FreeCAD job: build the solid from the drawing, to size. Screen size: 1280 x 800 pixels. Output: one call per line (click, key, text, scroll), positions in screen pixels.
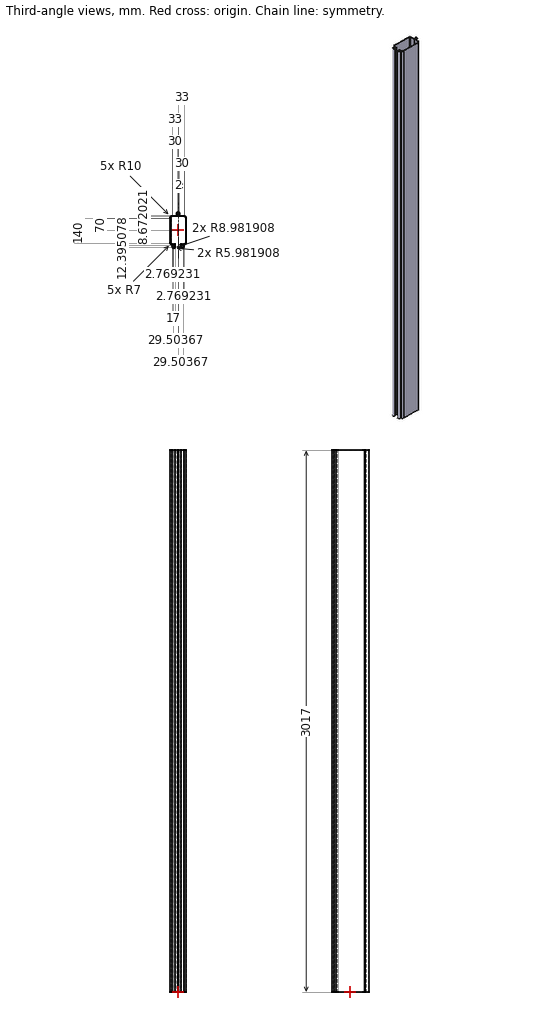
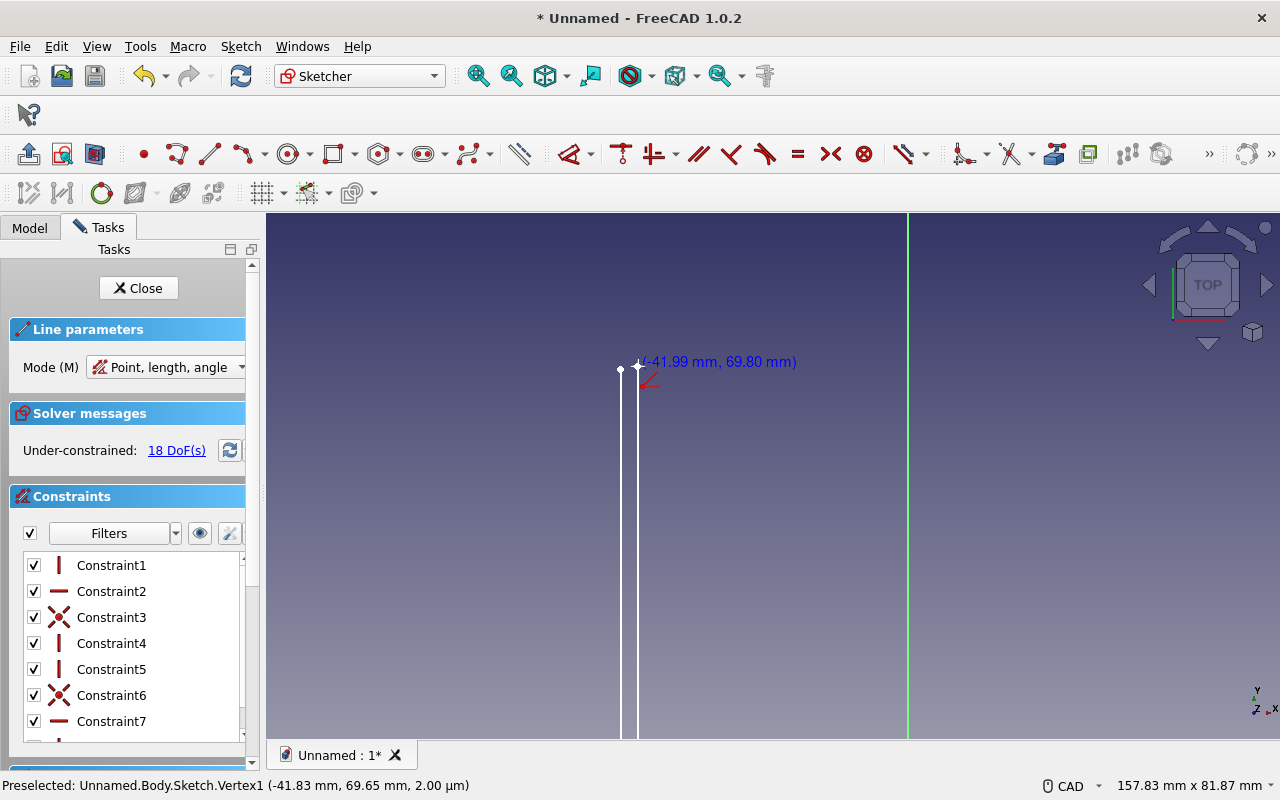
click(177, 154)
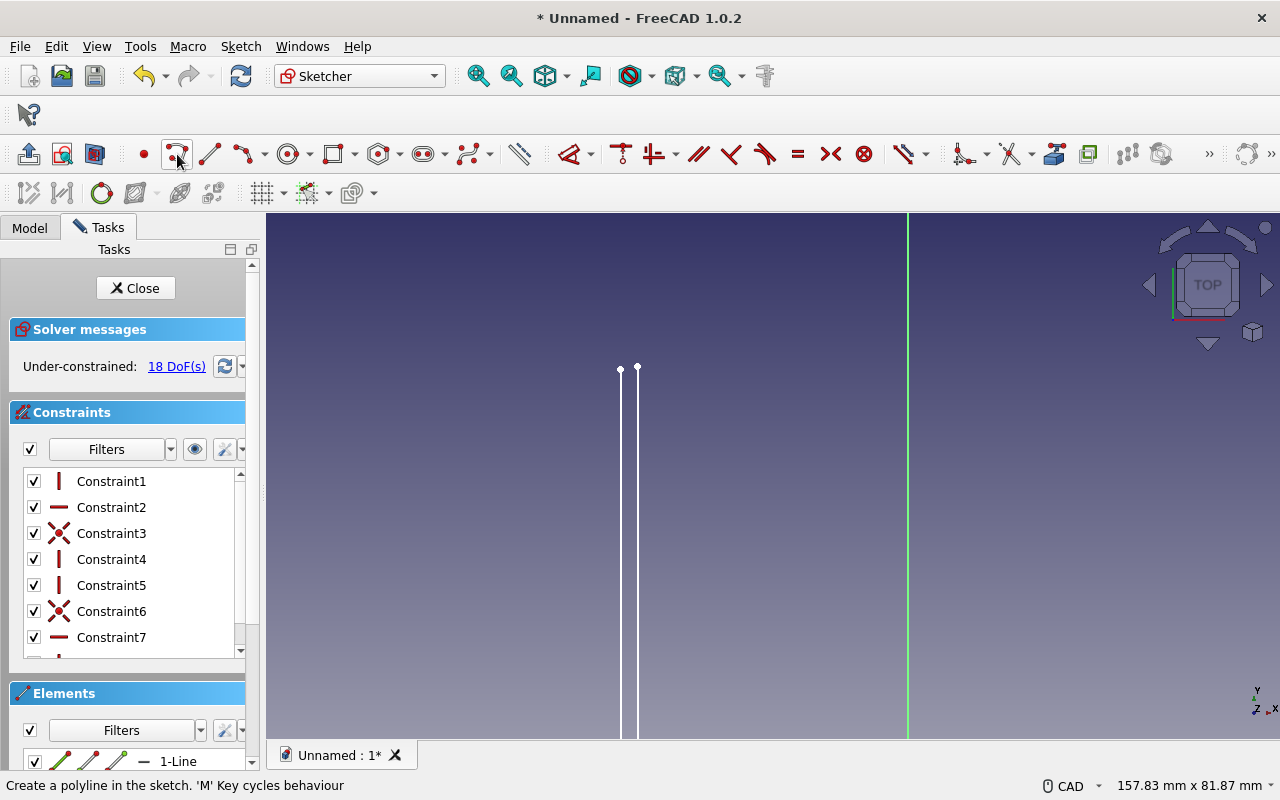
scroll(638, 366, down, 7)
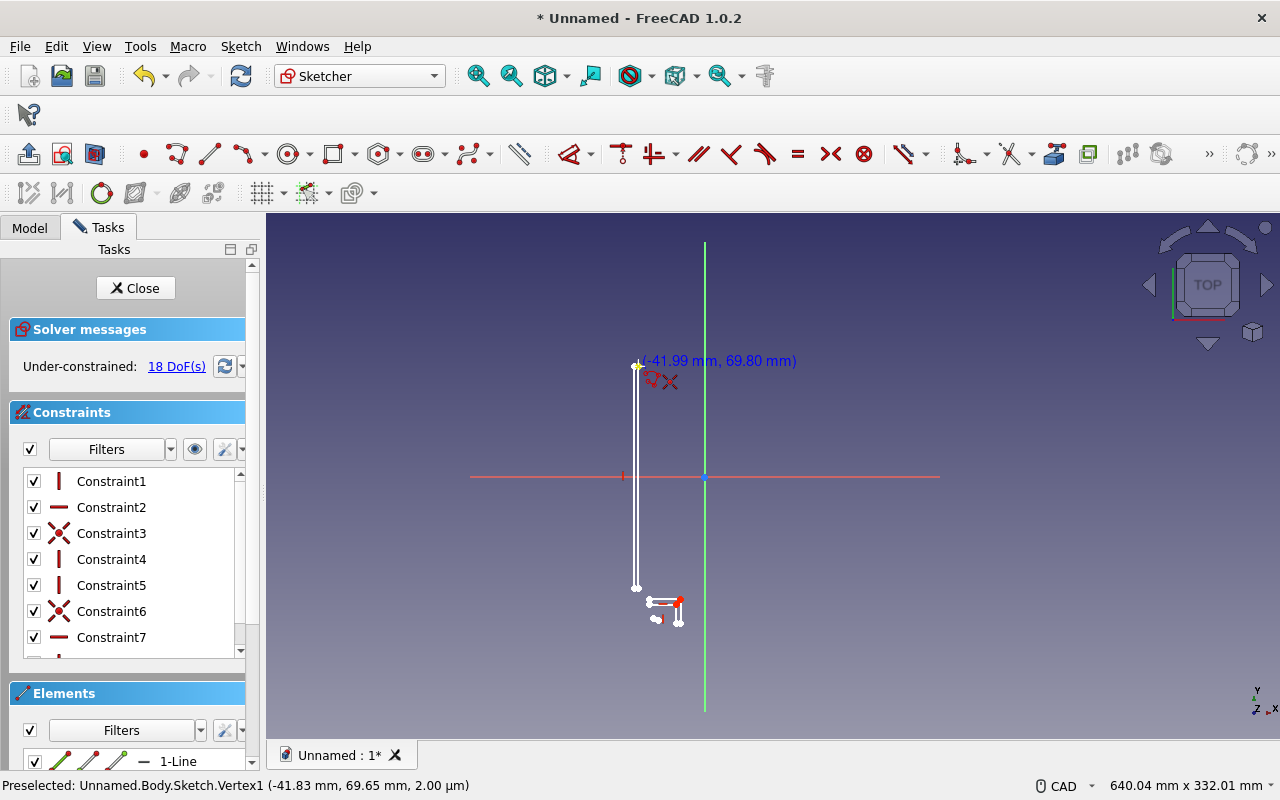
click(649, 355)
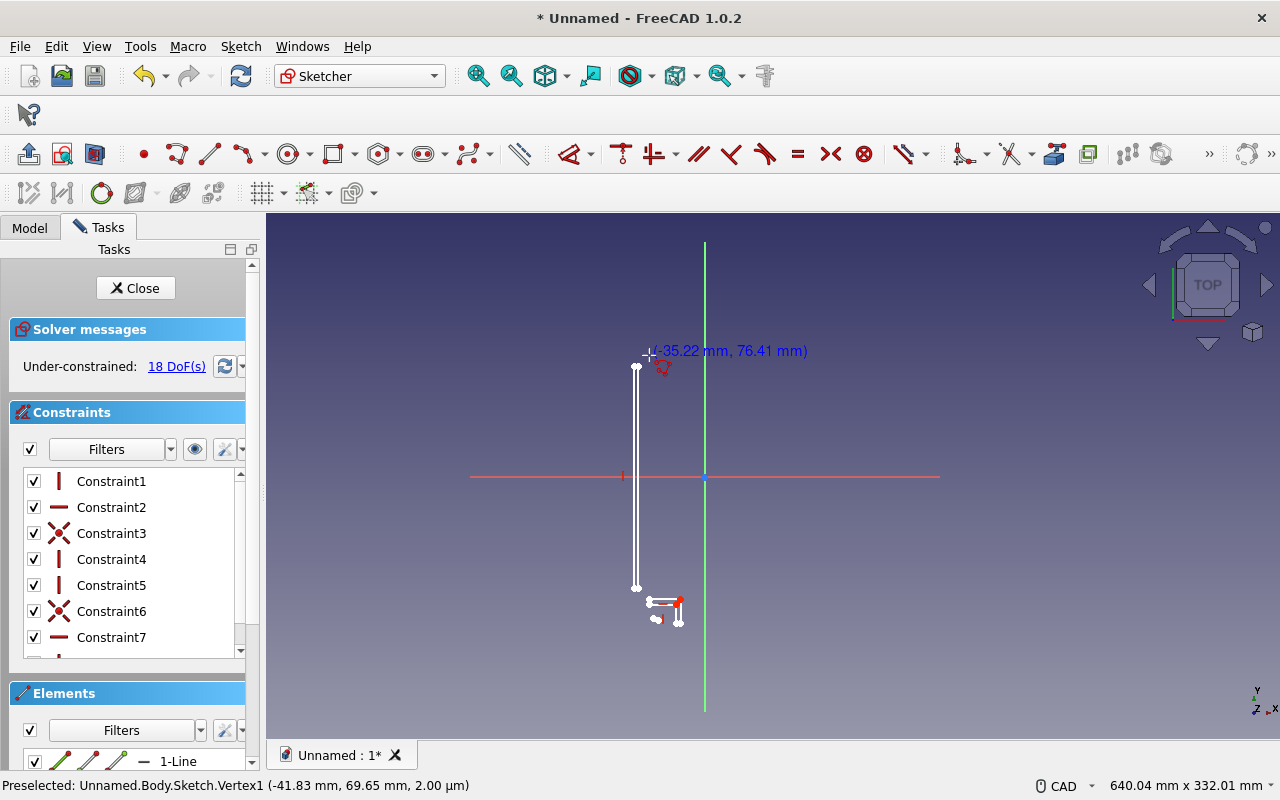
scroll(702, 355, up, 9)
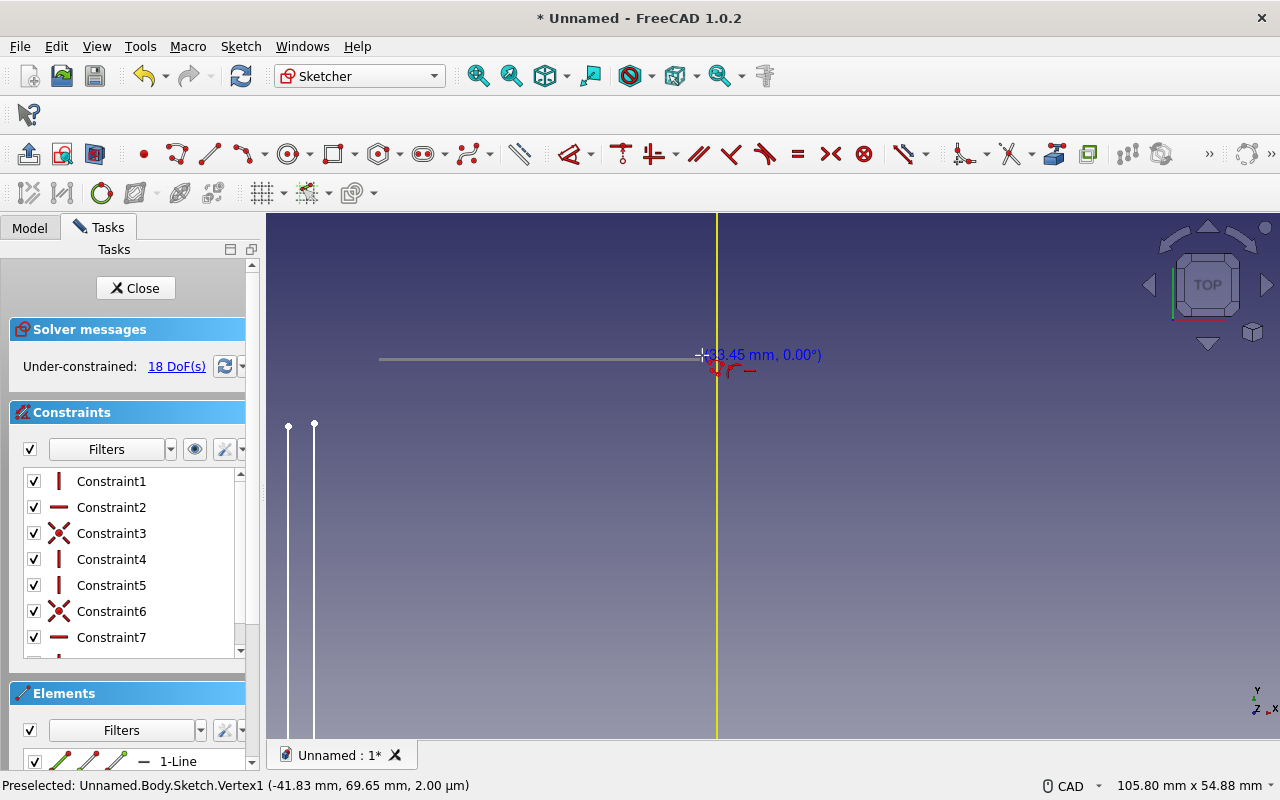
click(698, 354)
click(698, 271)
right_click(698, 271)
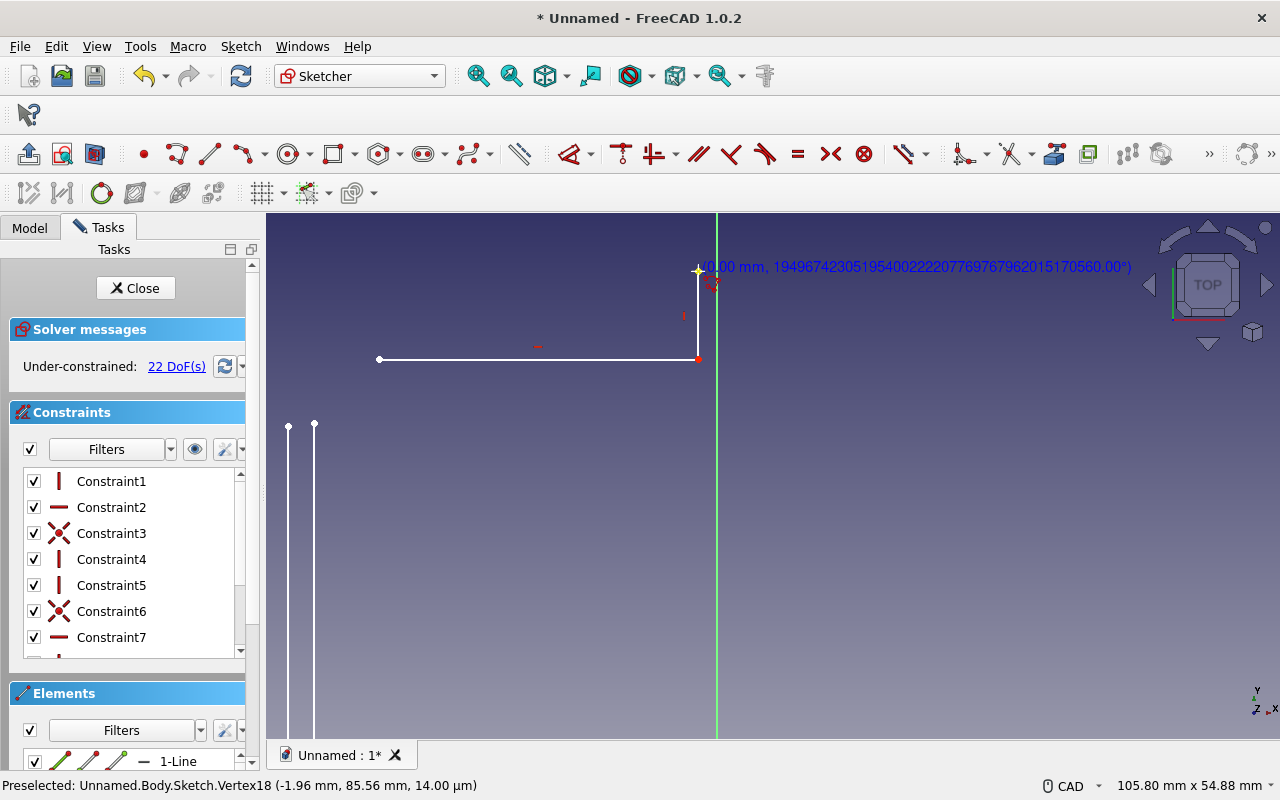
click(736, 271)
click(736, 354)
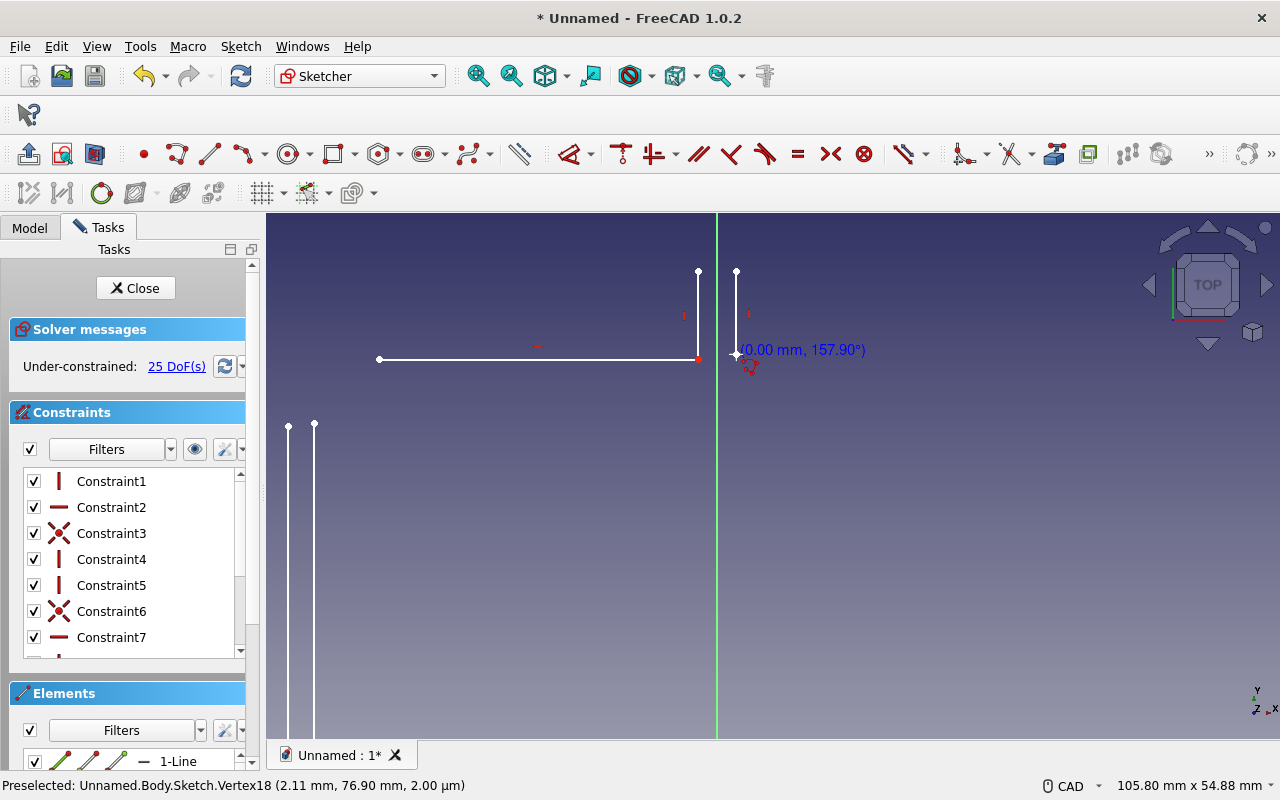
scroll(702, 355, down, 9)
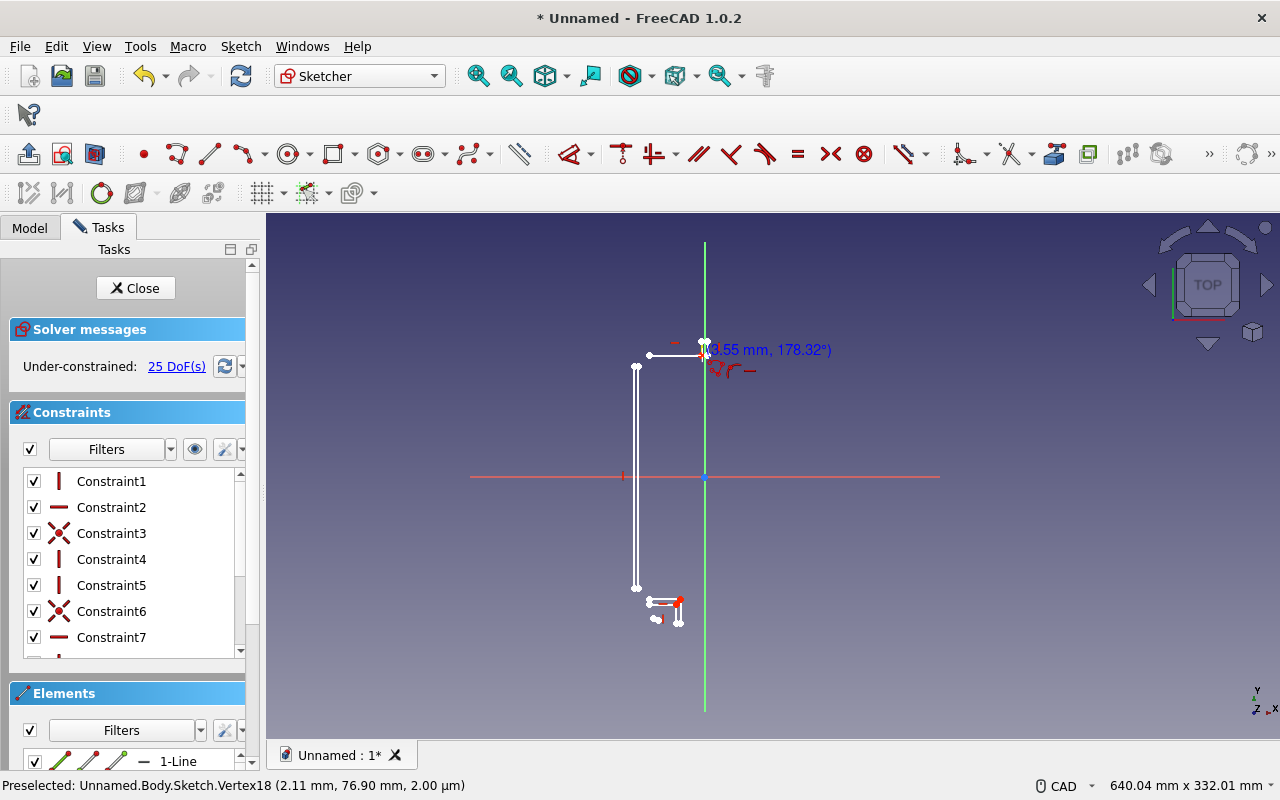
click(760, 355)
right_click(760, 355)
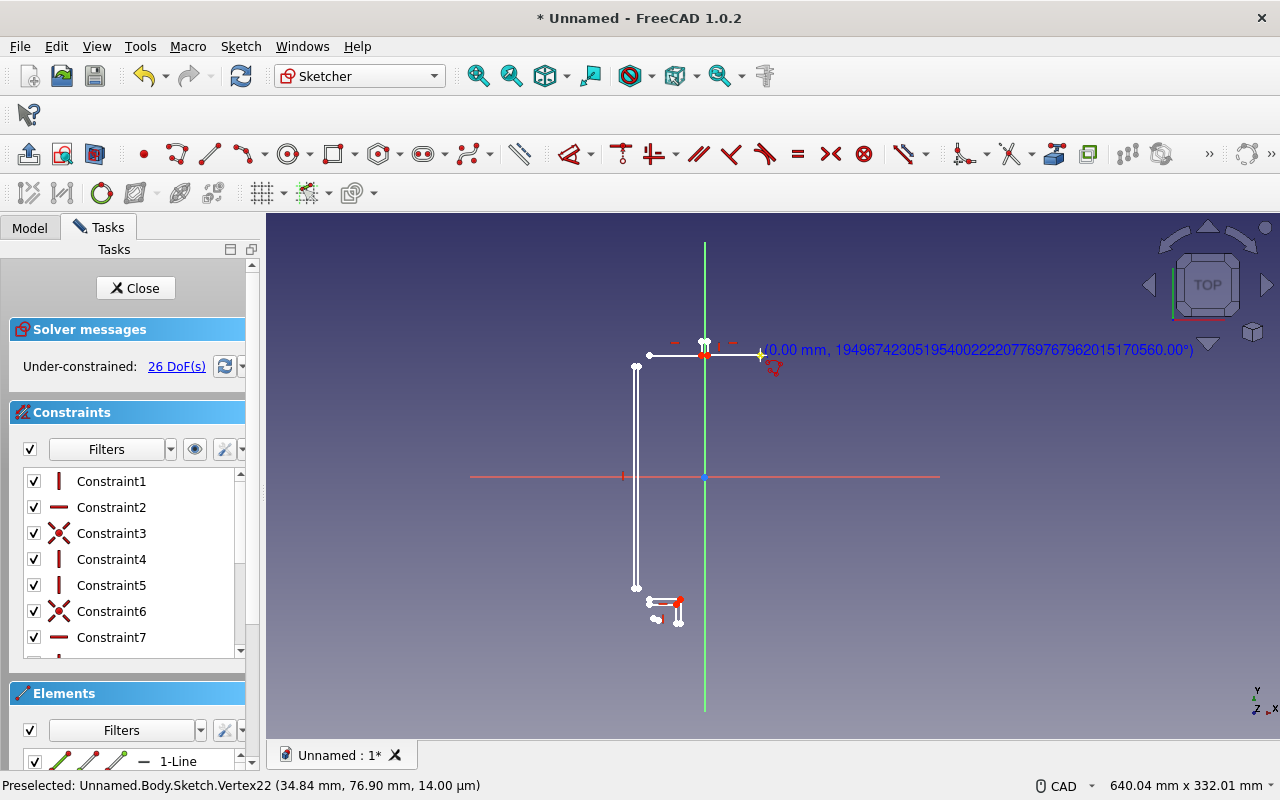
click(210, 154)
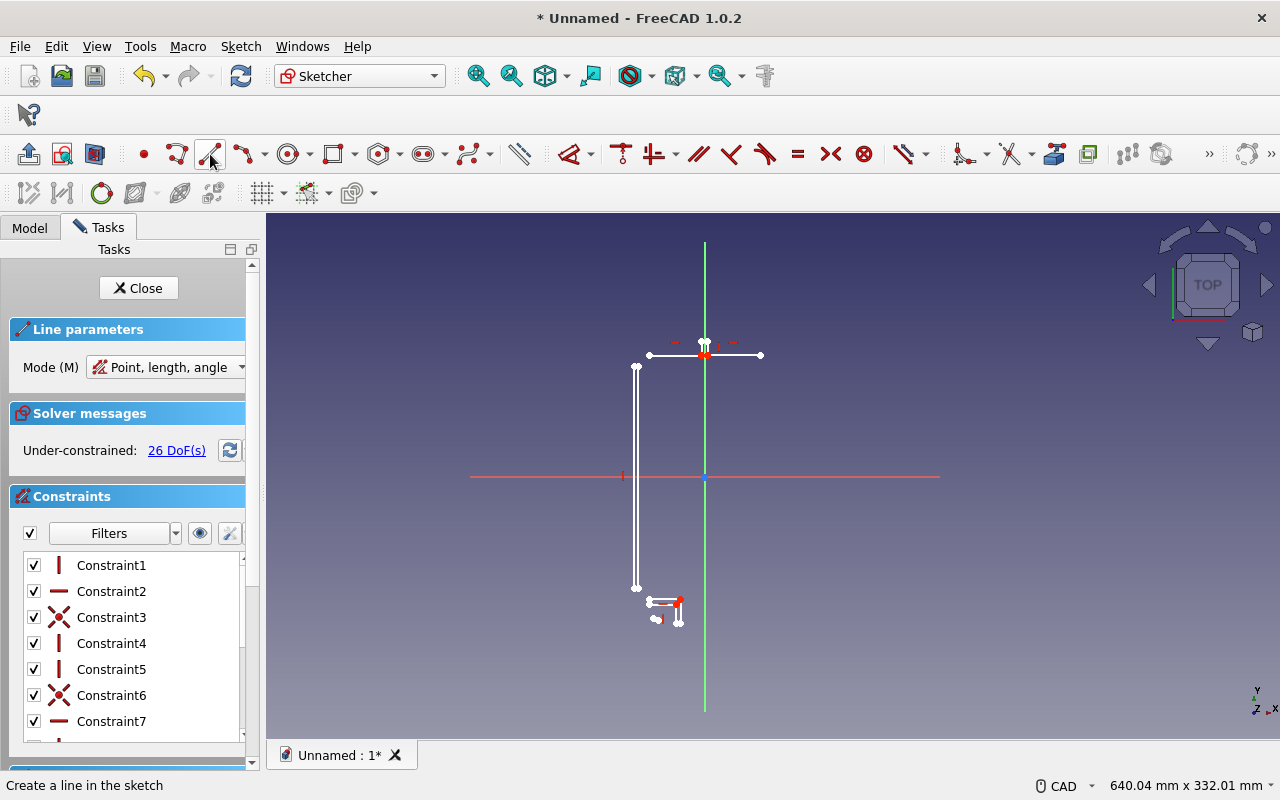
click(771, 366)
click(771, 588)